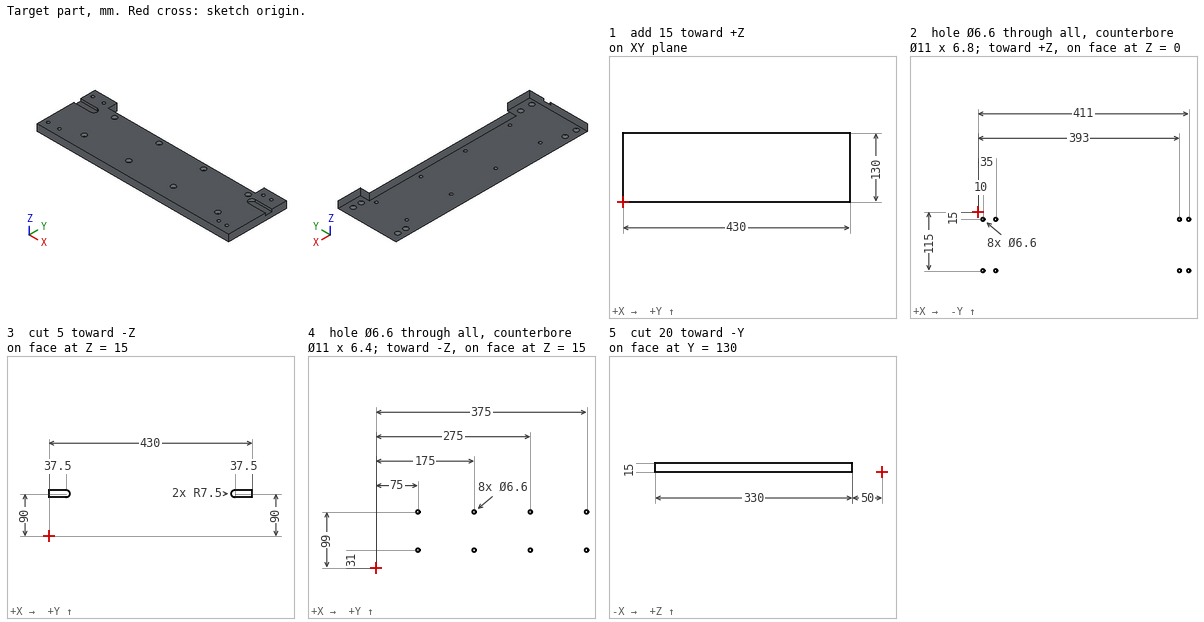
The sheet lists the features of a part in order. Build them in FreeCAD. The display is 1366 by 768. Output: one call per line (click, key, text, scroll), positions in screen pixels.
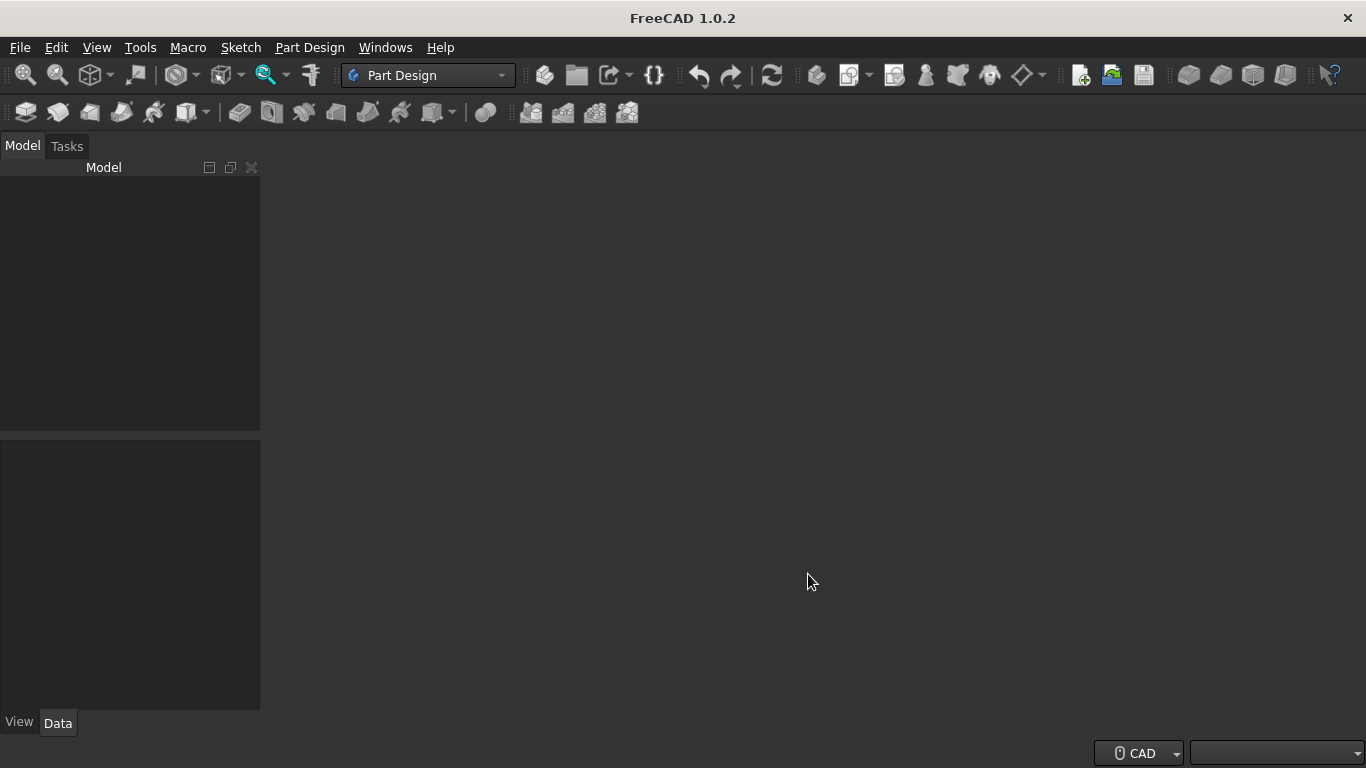
click(1080, 76)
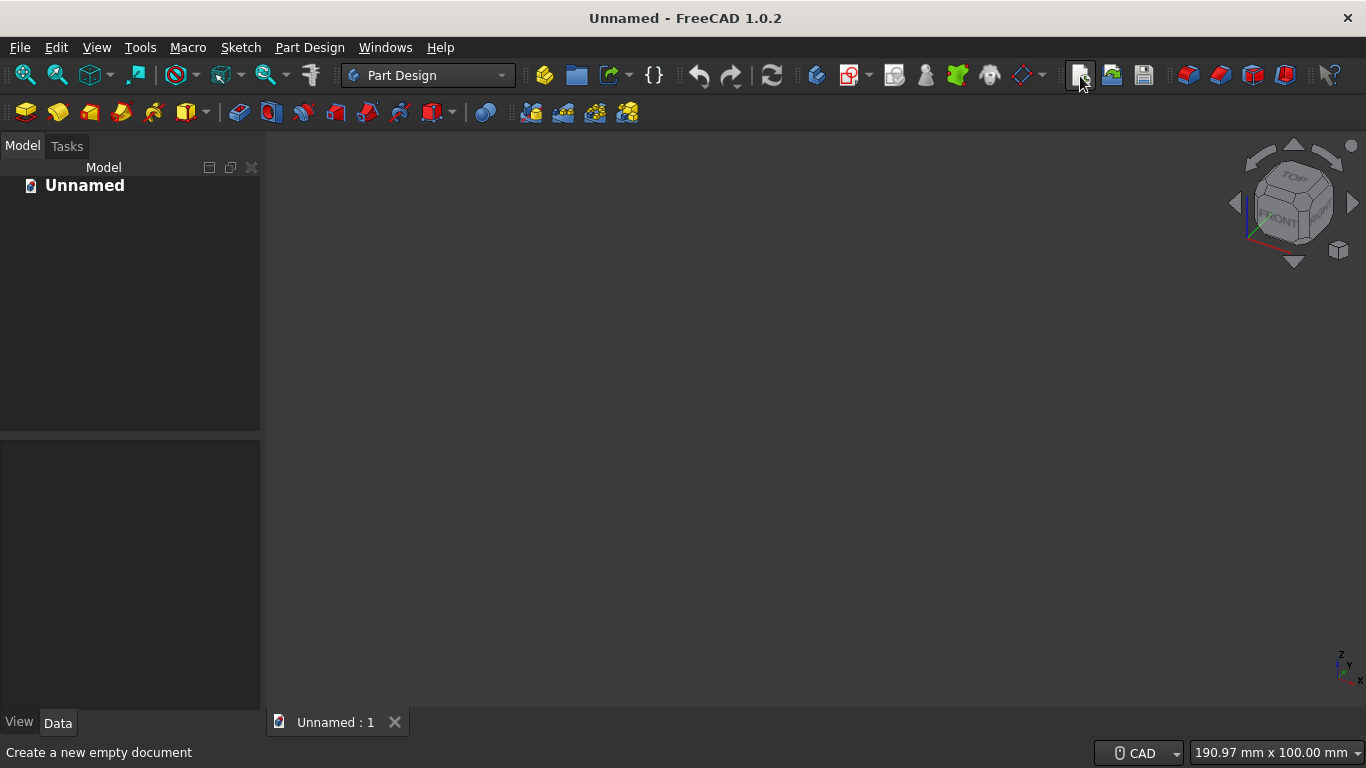
click(850, 76)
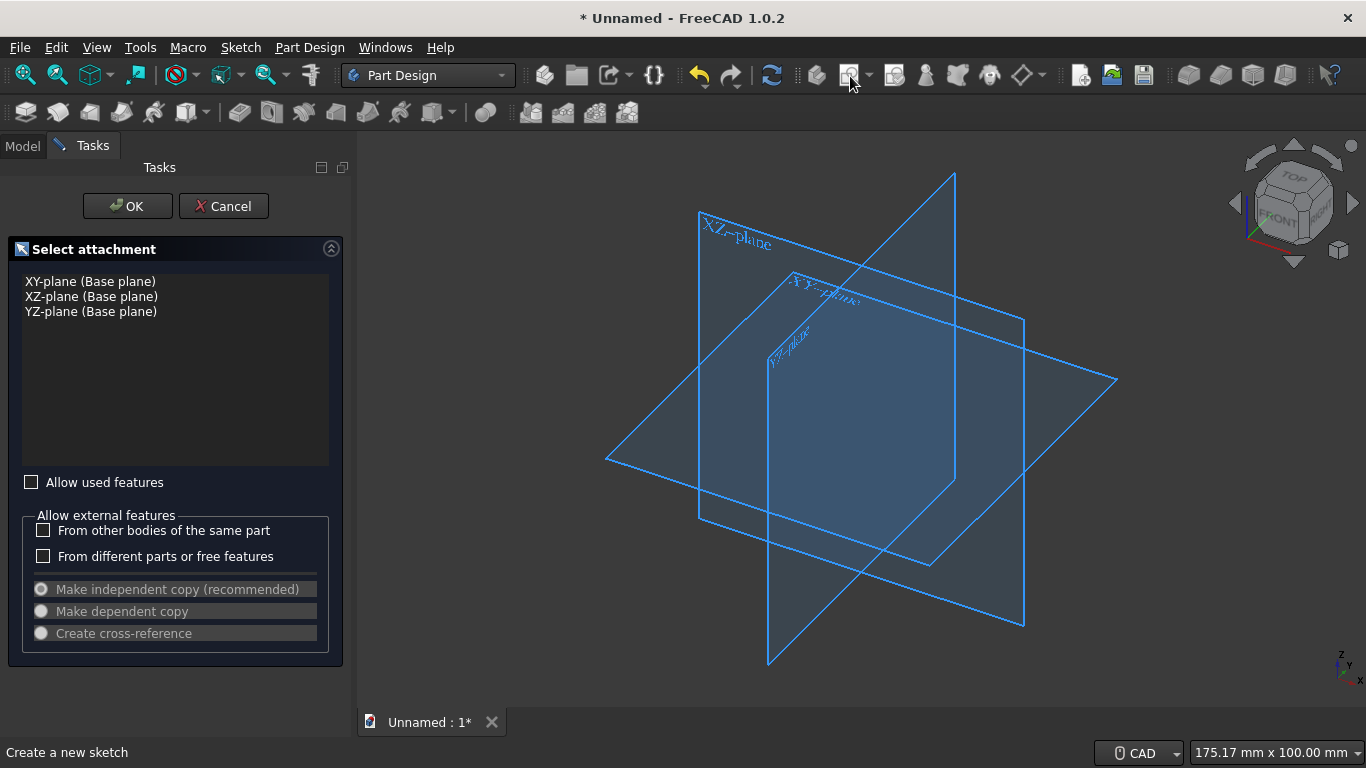
click(82, 282)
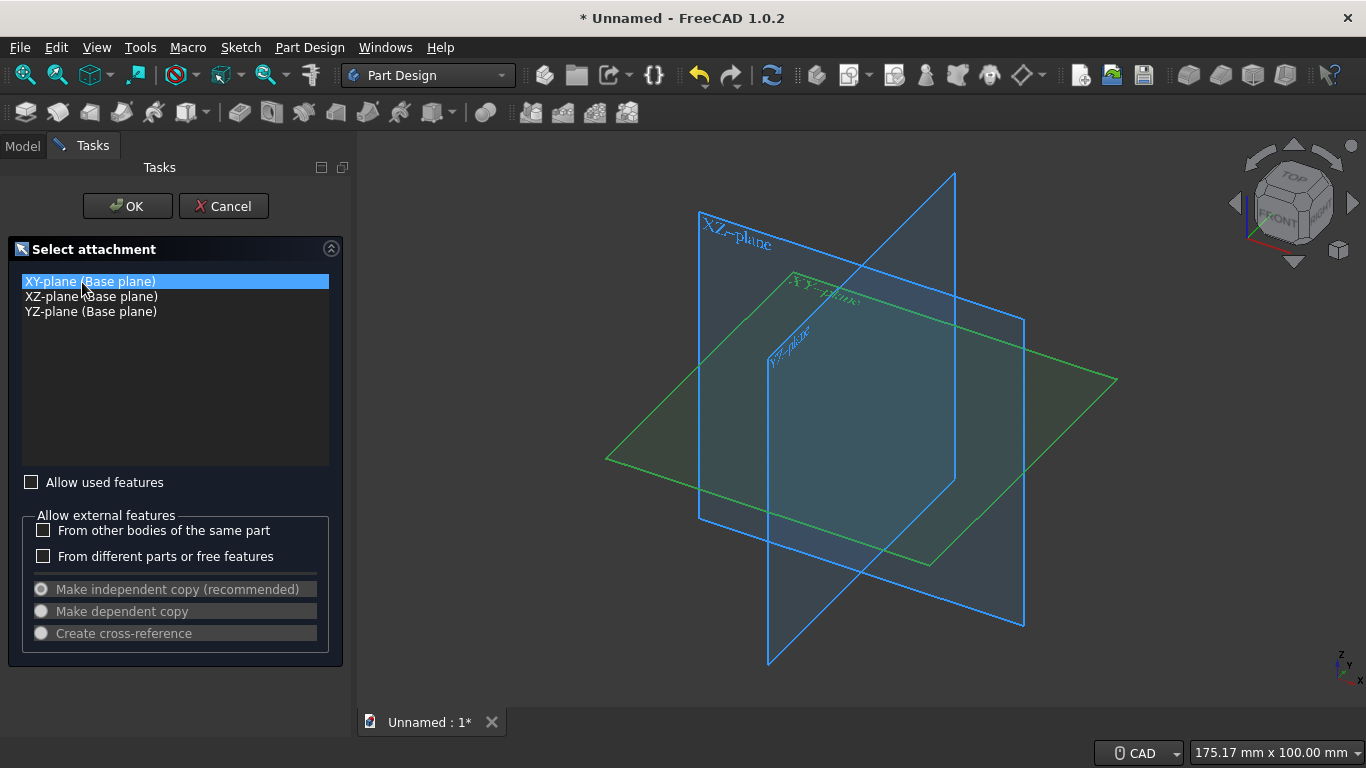
click(128, 206)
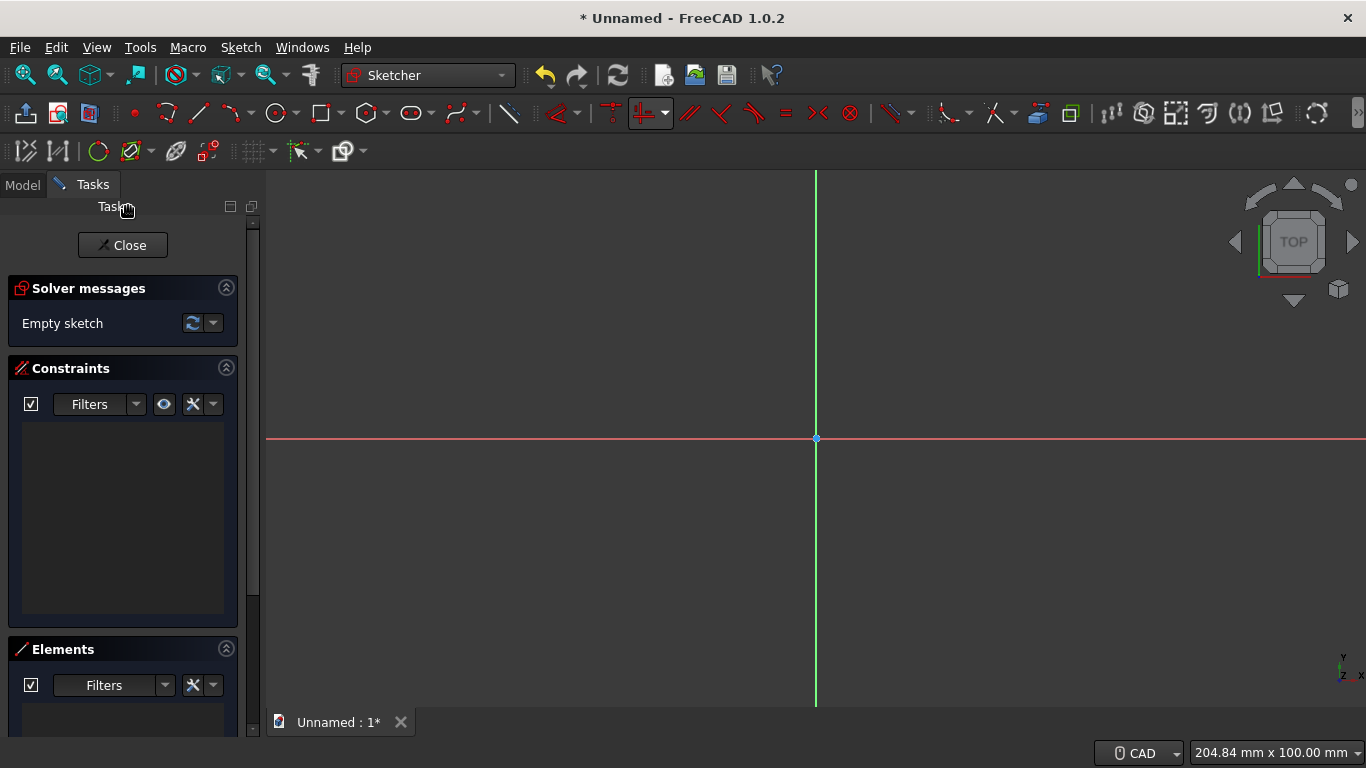
scroll(294, 589, down, 6)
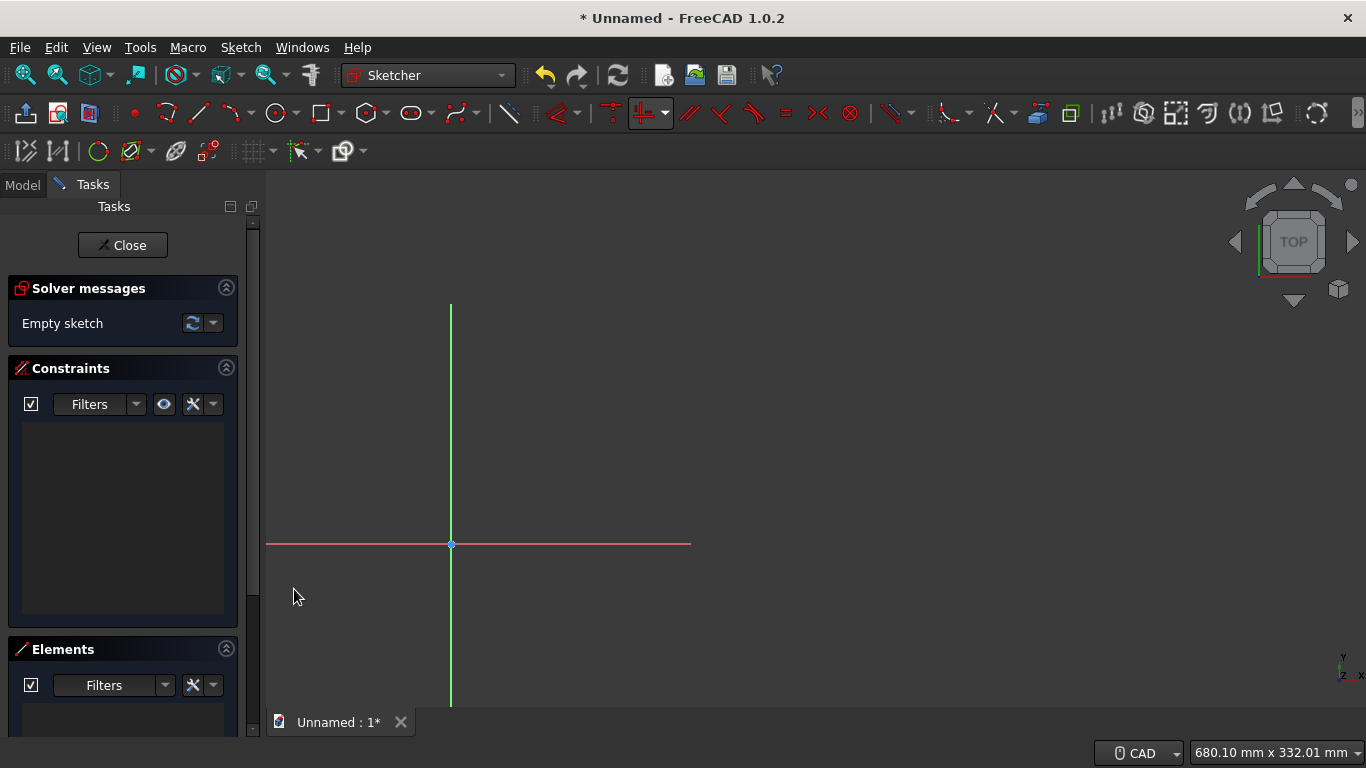
click(322, 114)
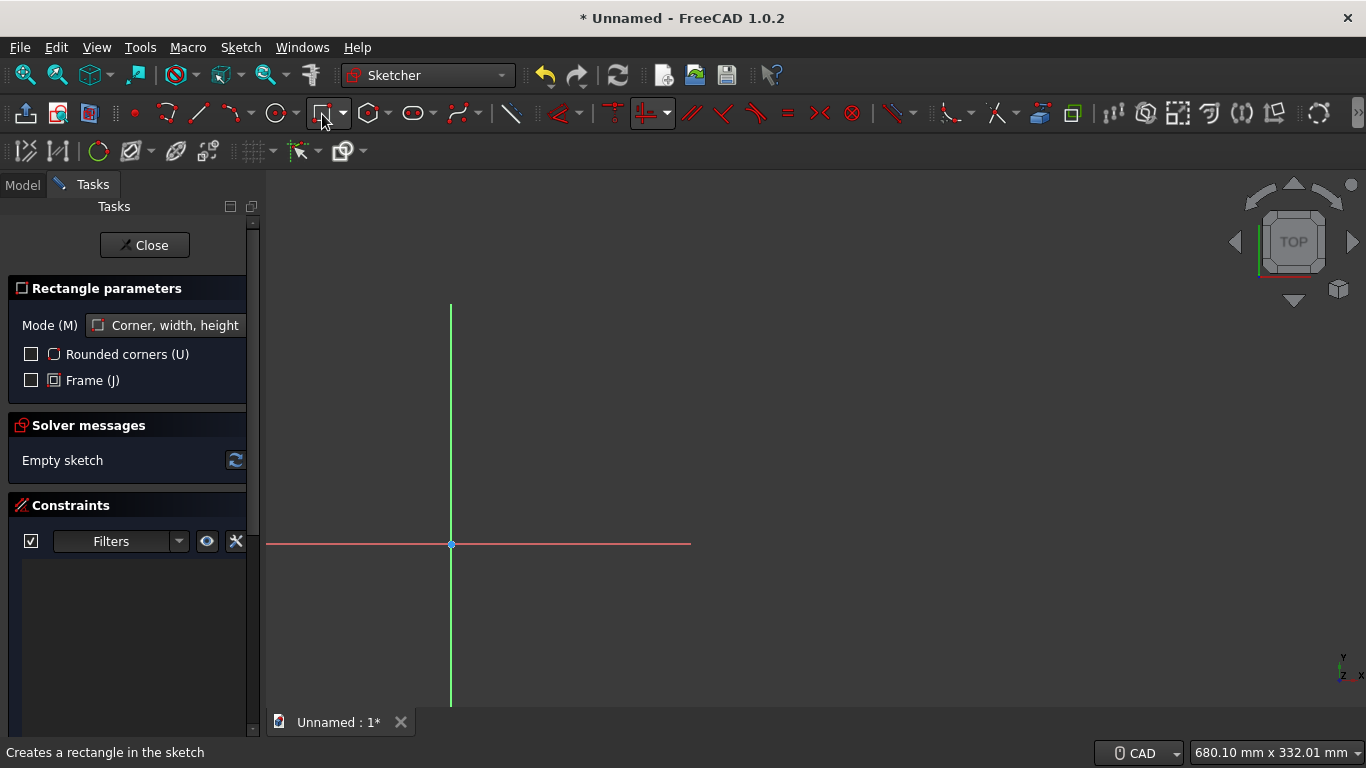
click(451, 544)
click(1147, 334)
key(Escape)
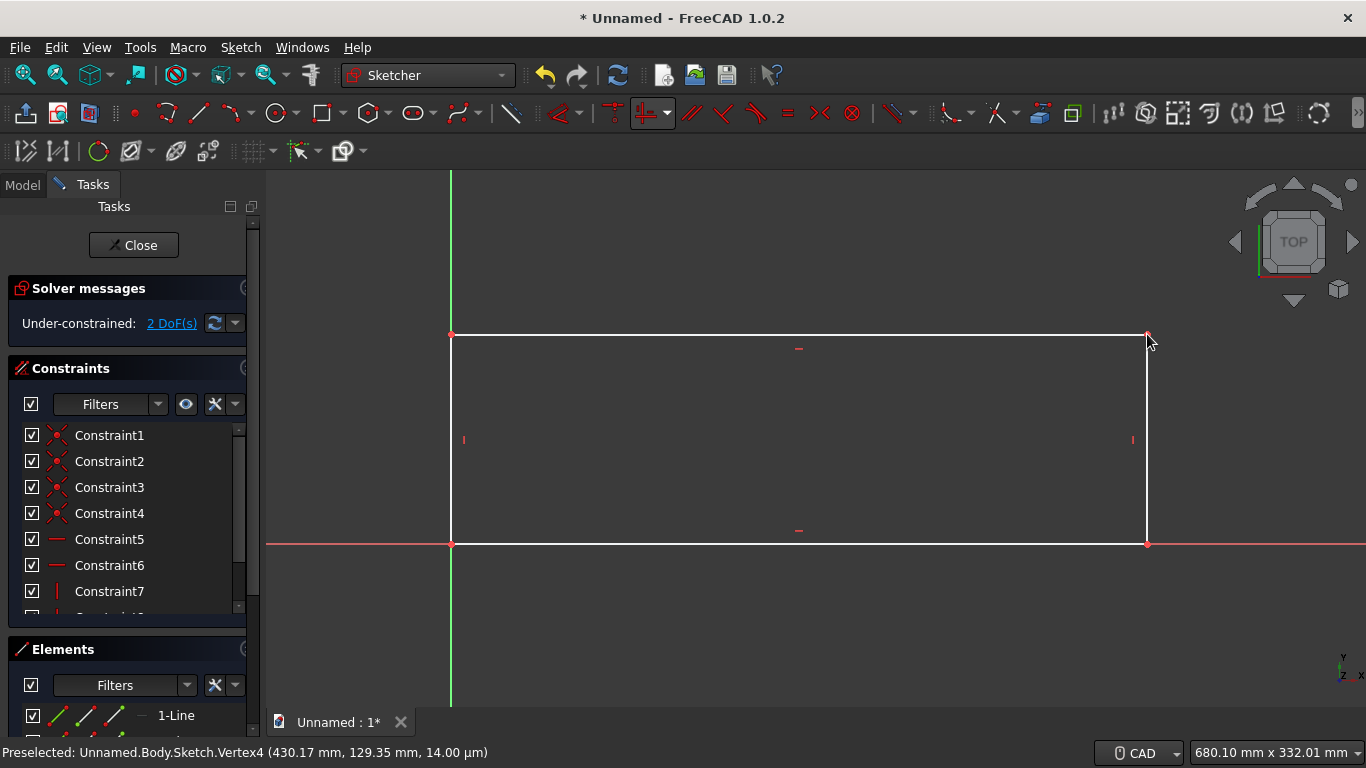
click(660, 544)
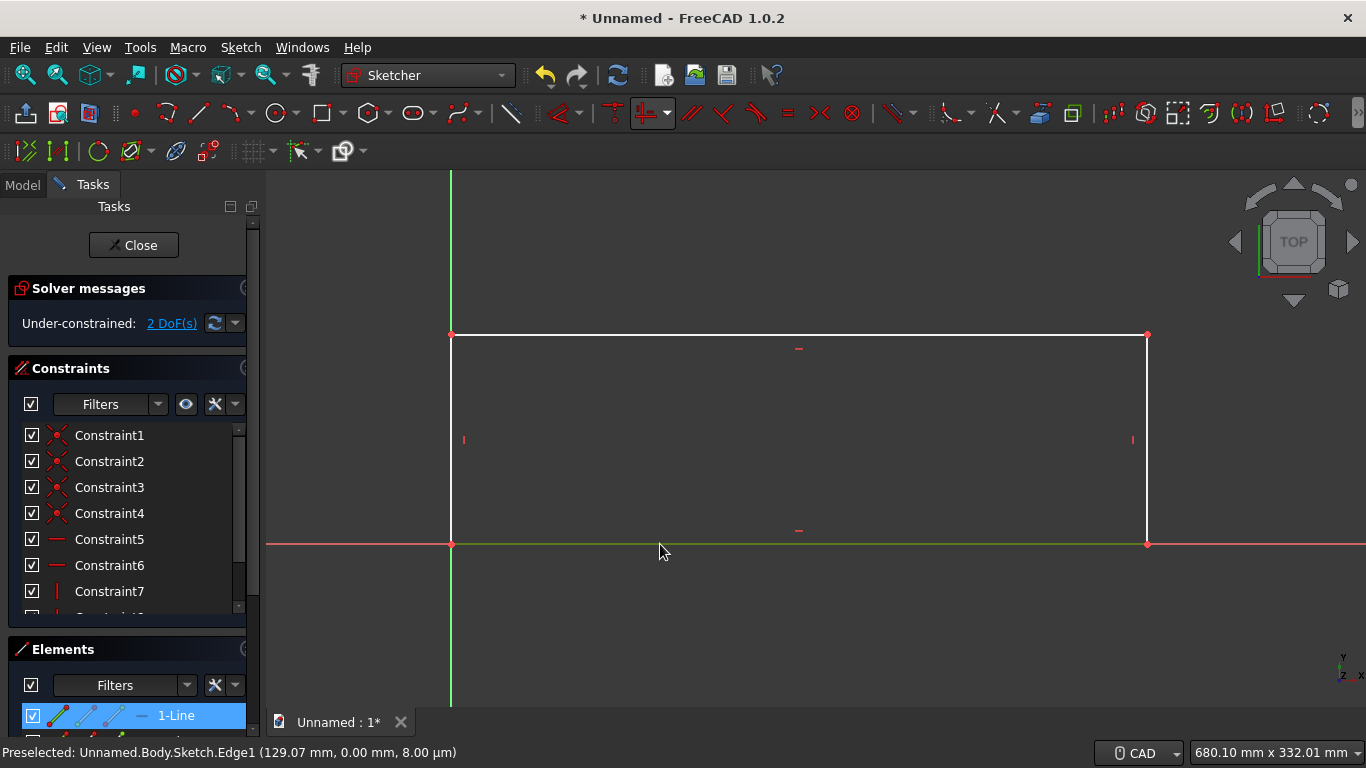
key(l)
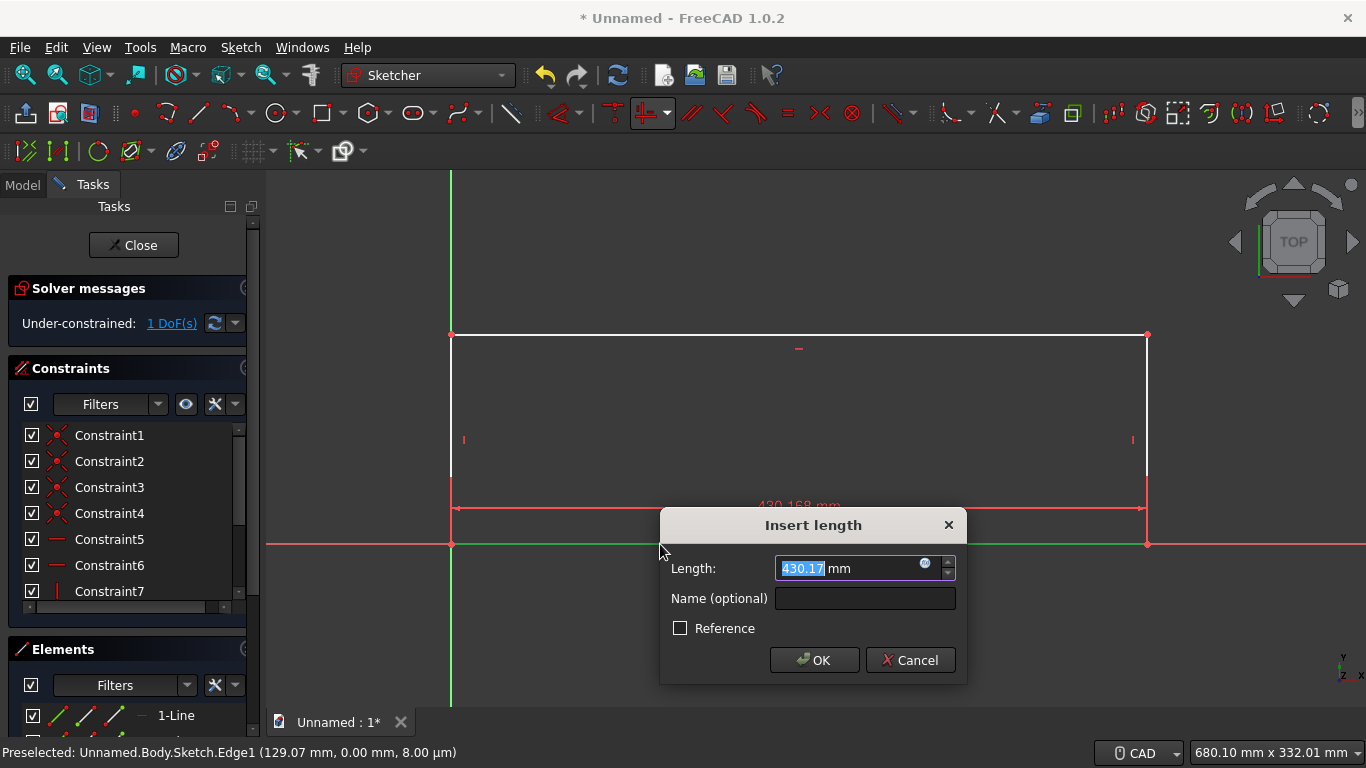
text(430)
key(Return)